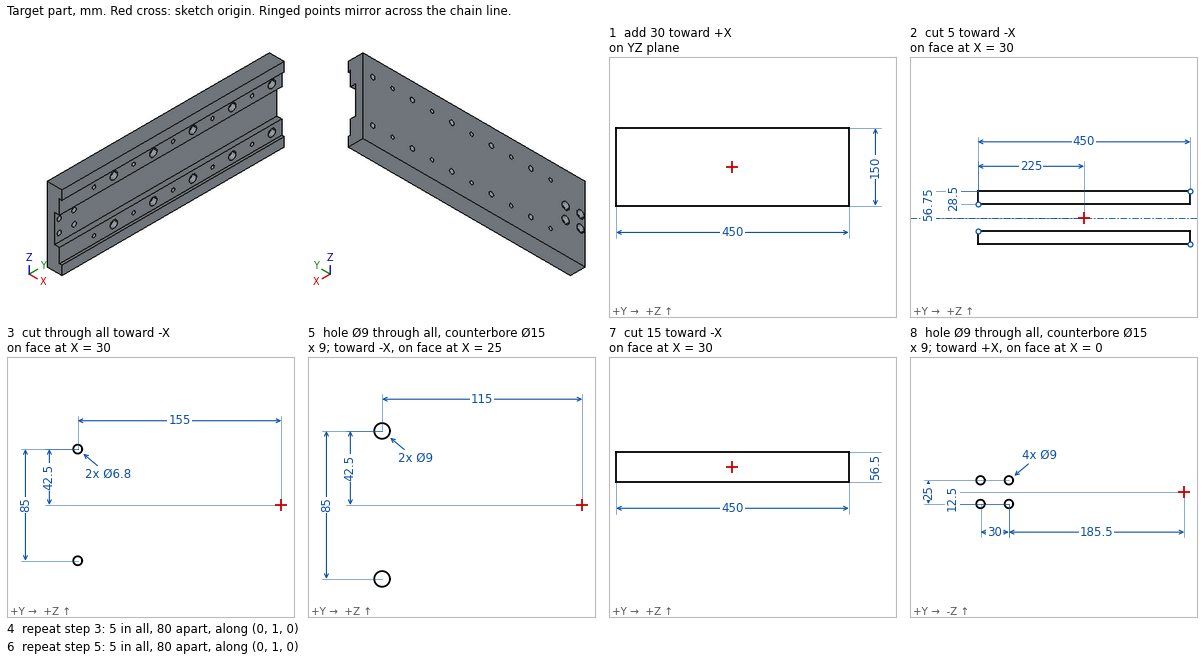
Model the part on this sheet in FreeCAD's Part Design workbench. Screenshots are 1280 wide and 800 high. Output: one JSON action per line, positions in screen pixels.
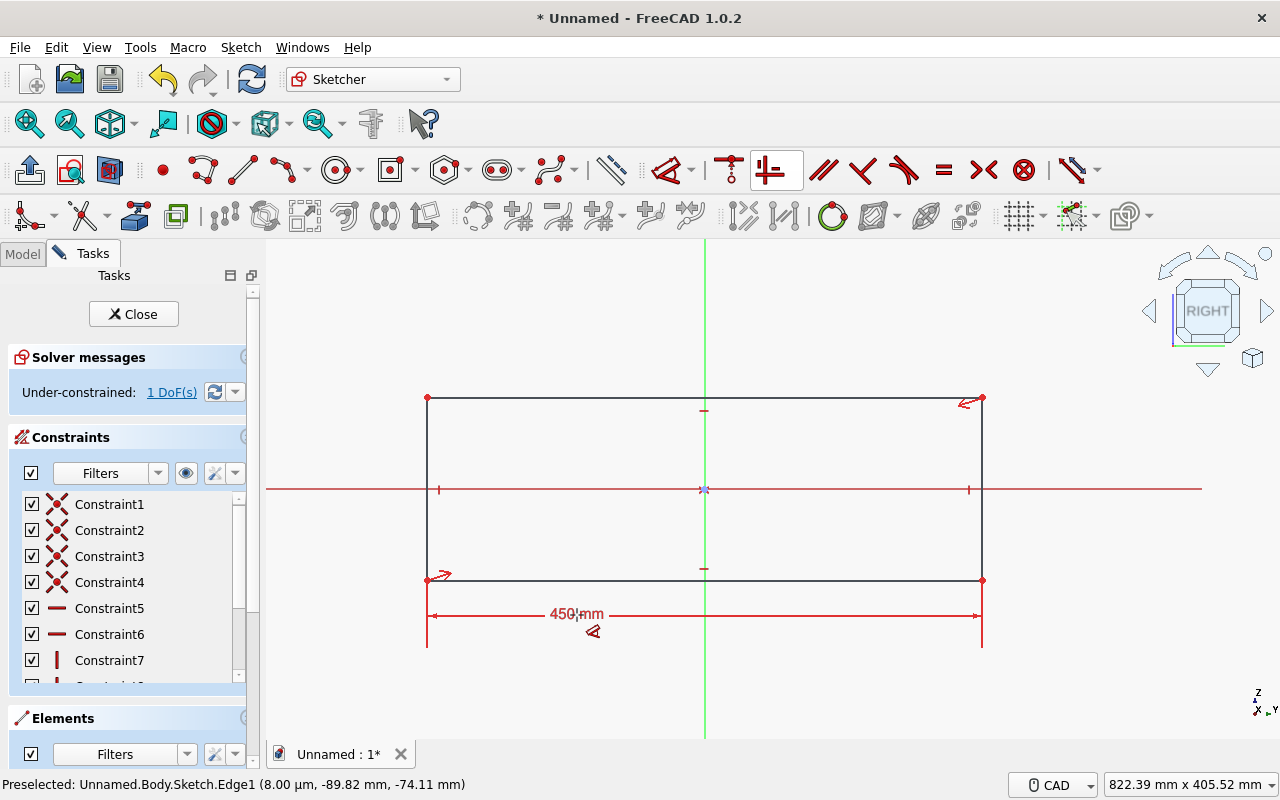
{"action": "left_click", "coordinate": [982, 526]}
{"action": "left_click", "coordinate": [1016, 447]}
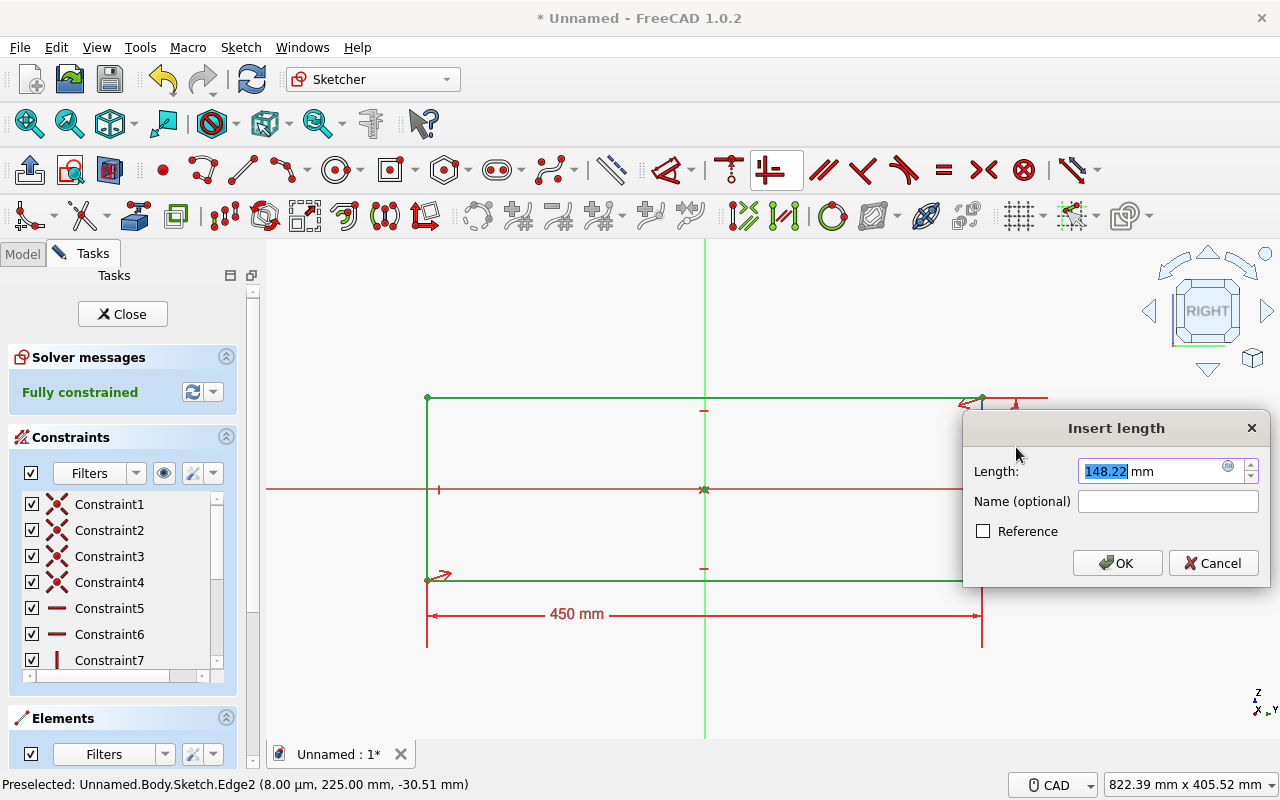
{"action": "type", "text": "150"}
{"action": "key", "text": "Return"}
{"action": "key", "text": "Escape"}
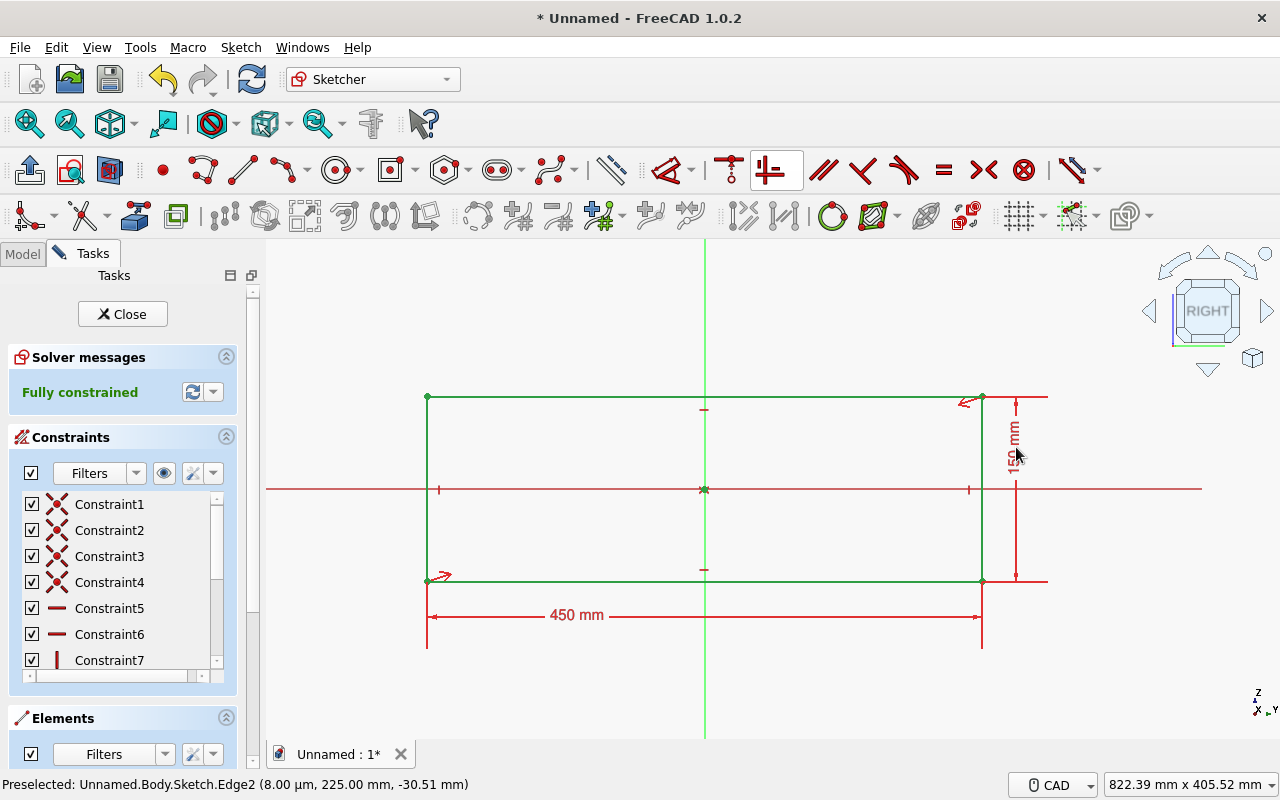
{"action": "left_click", "coordinate": [123, 314]}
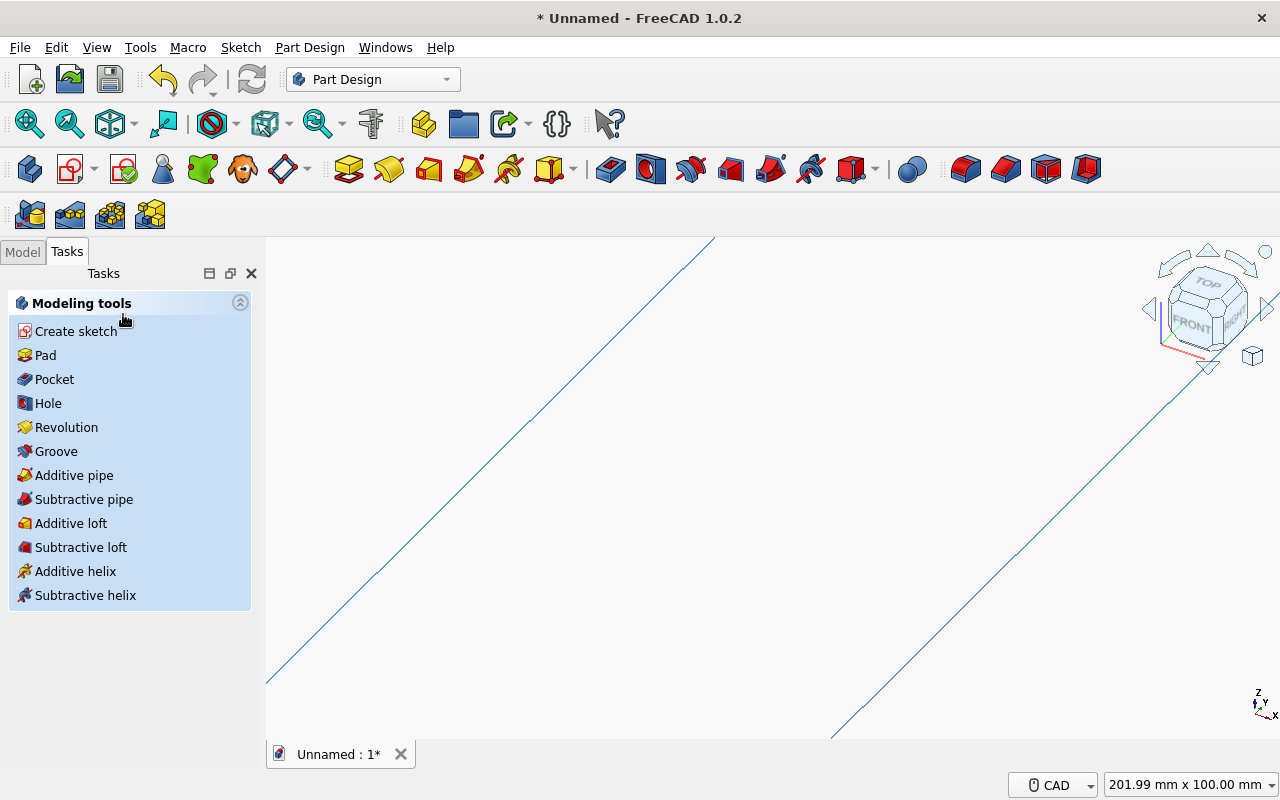
{"action": "left_click", "coordinate": [350, 170]}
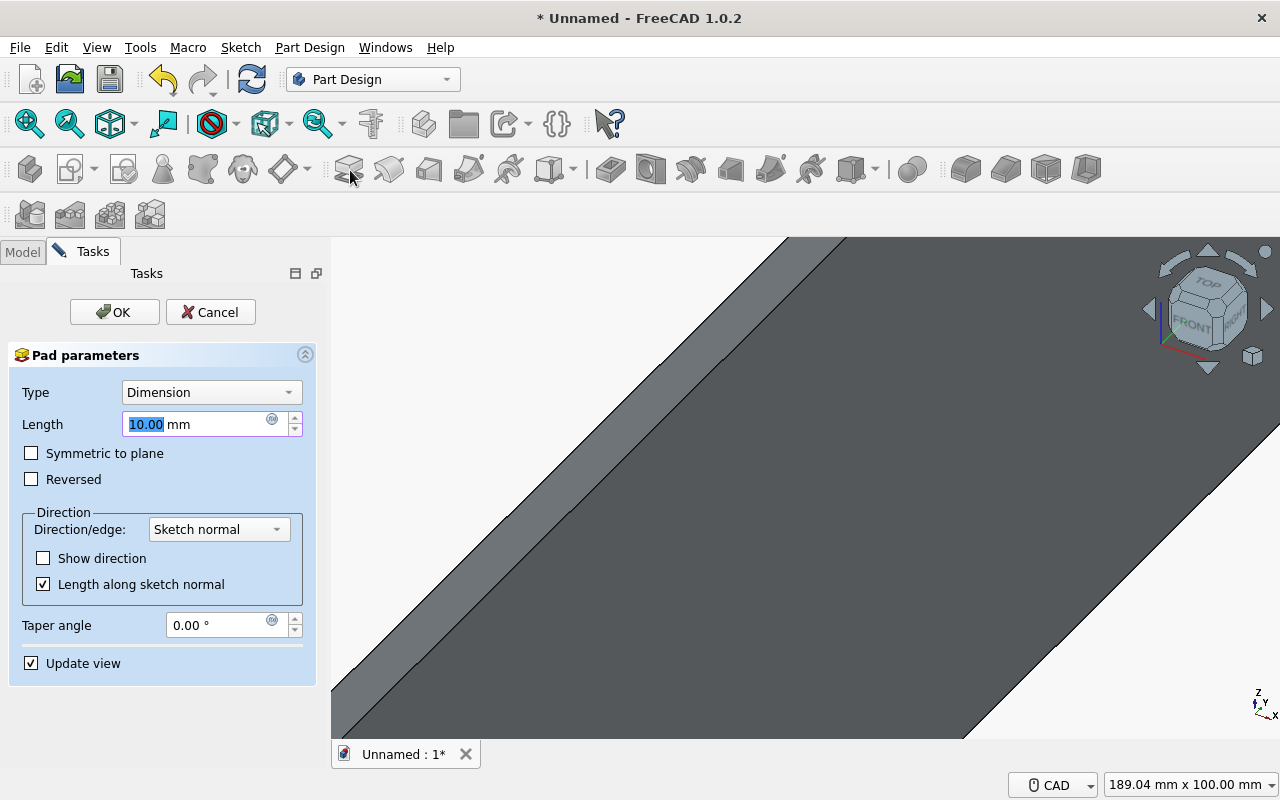
{"action": "type", "text": "30"}
{"action": "key", "text": "Tab"}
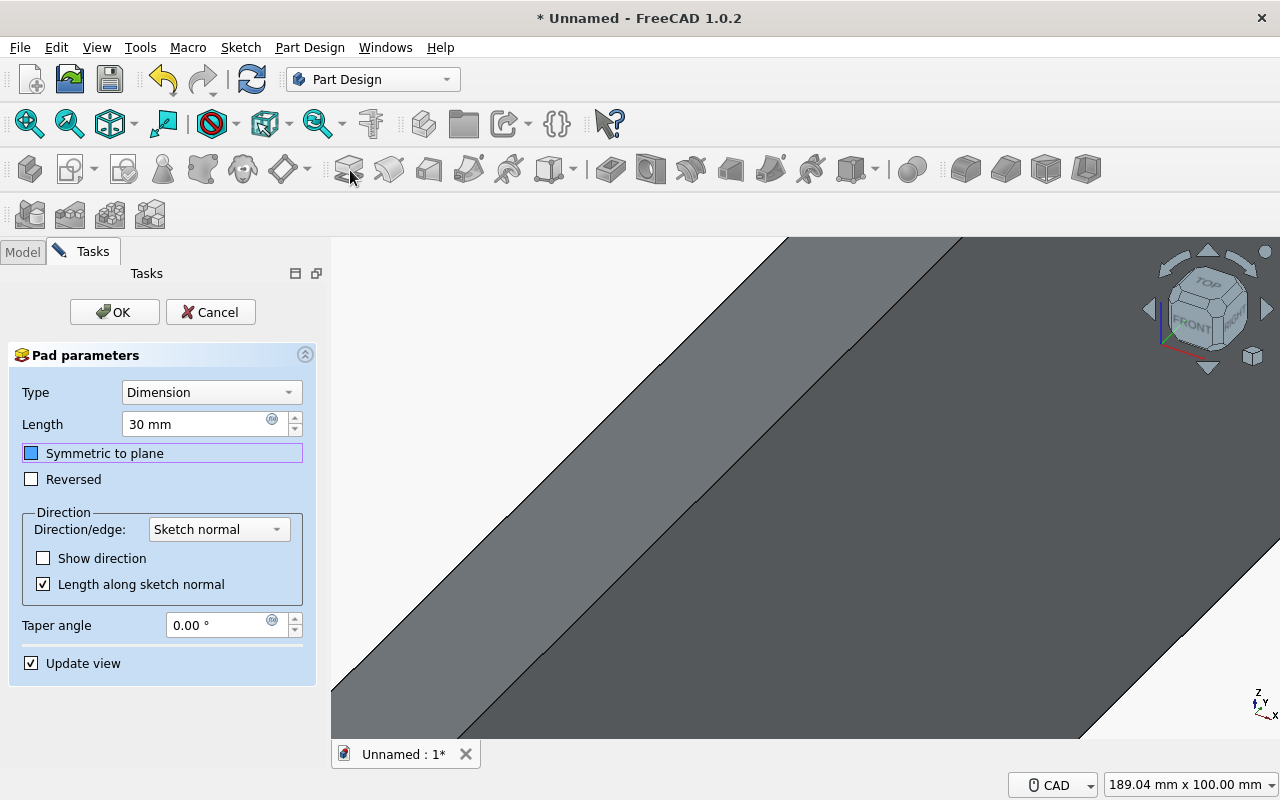
{"action": "left_click", "coordinate": [115, 312]}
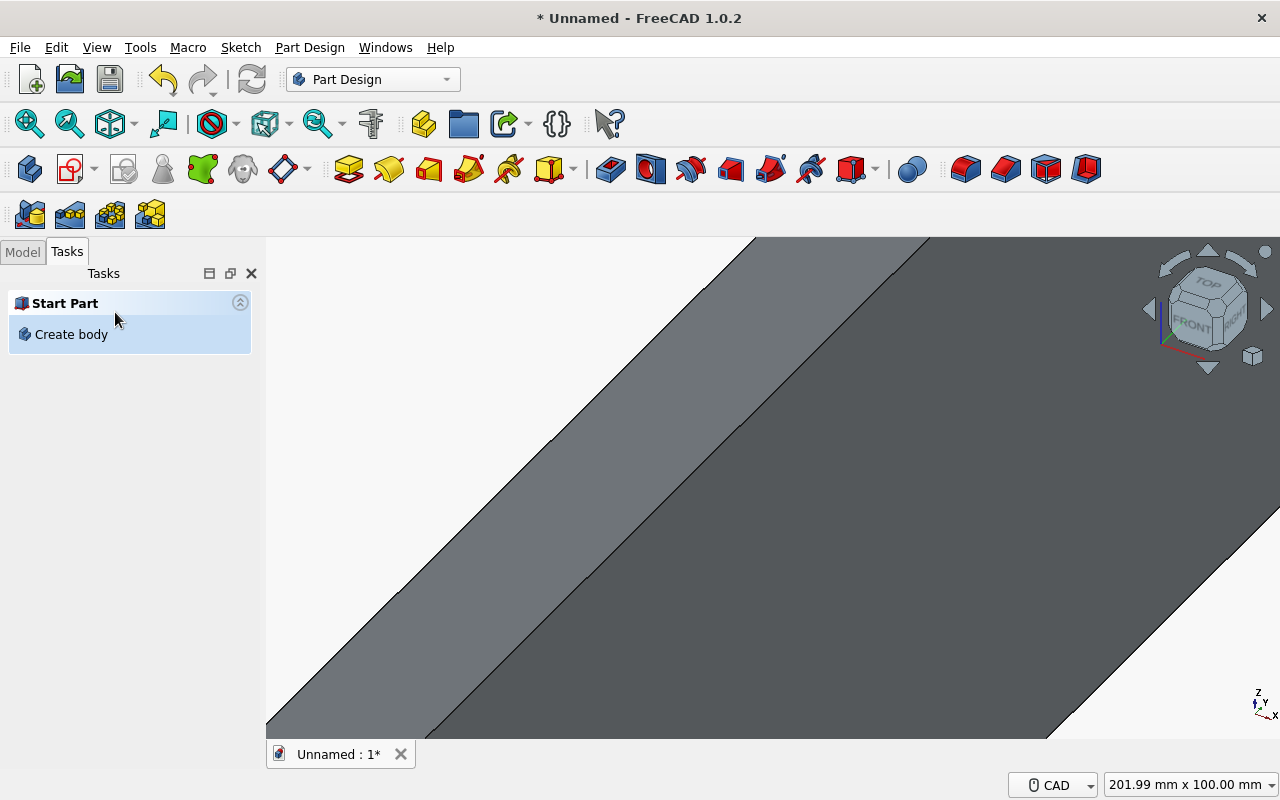
{"action": "left_click", "coordinate": [30, 124]}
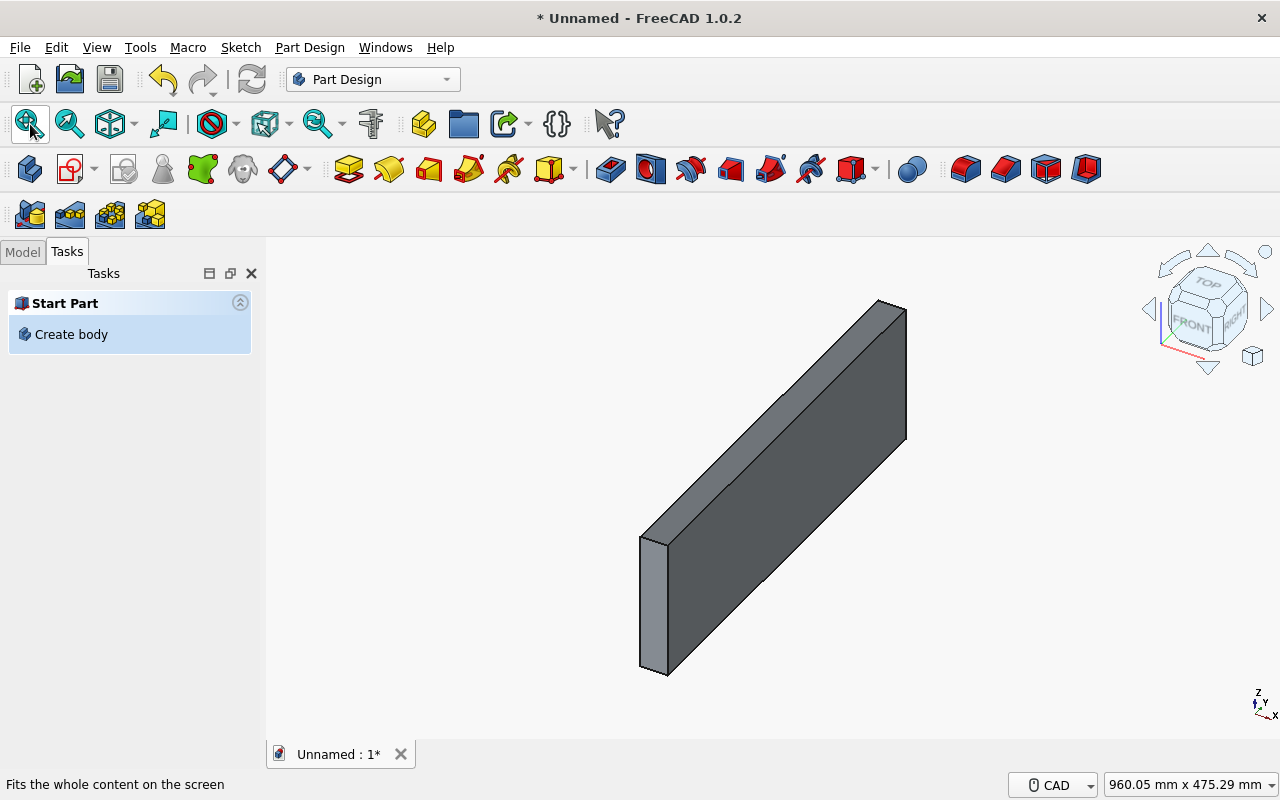
{"action": "left_click", "coordinate": [855, 424]}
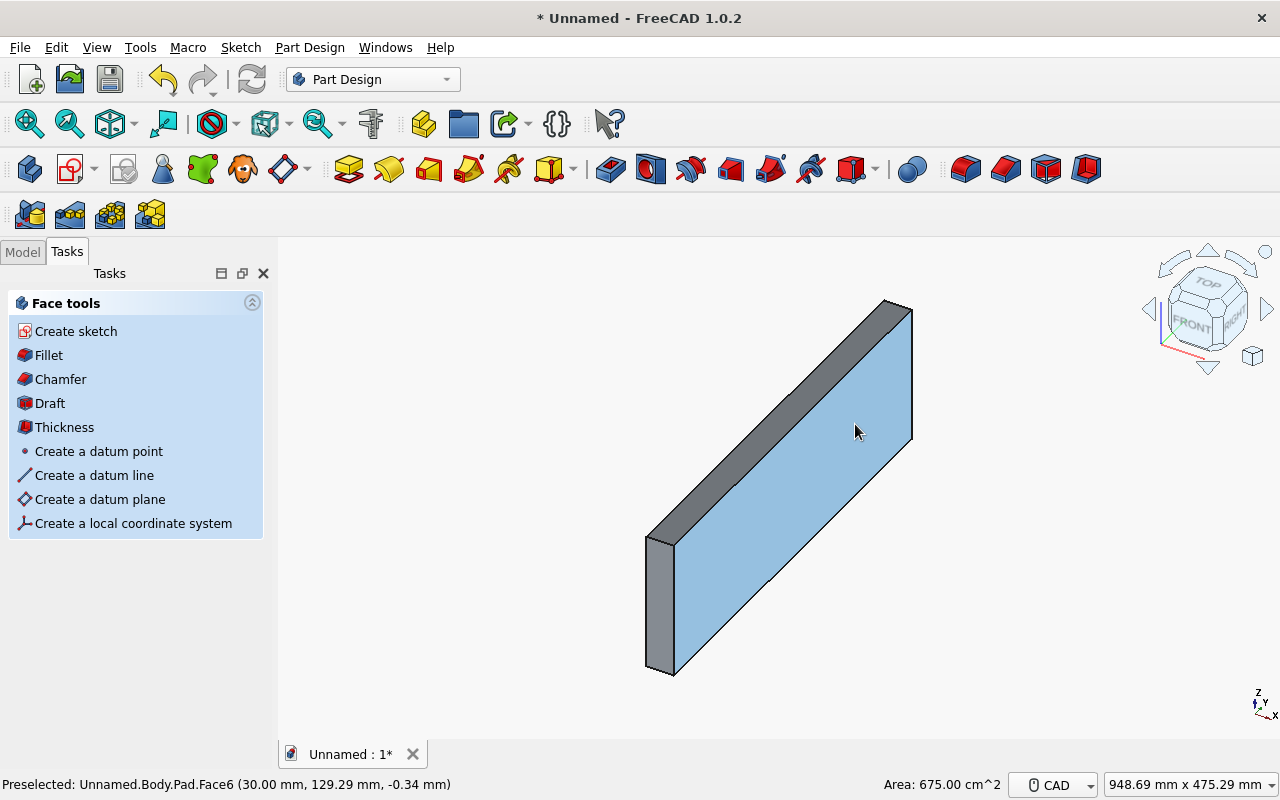
{"action": "left_click", "coordinate": [70, 170]}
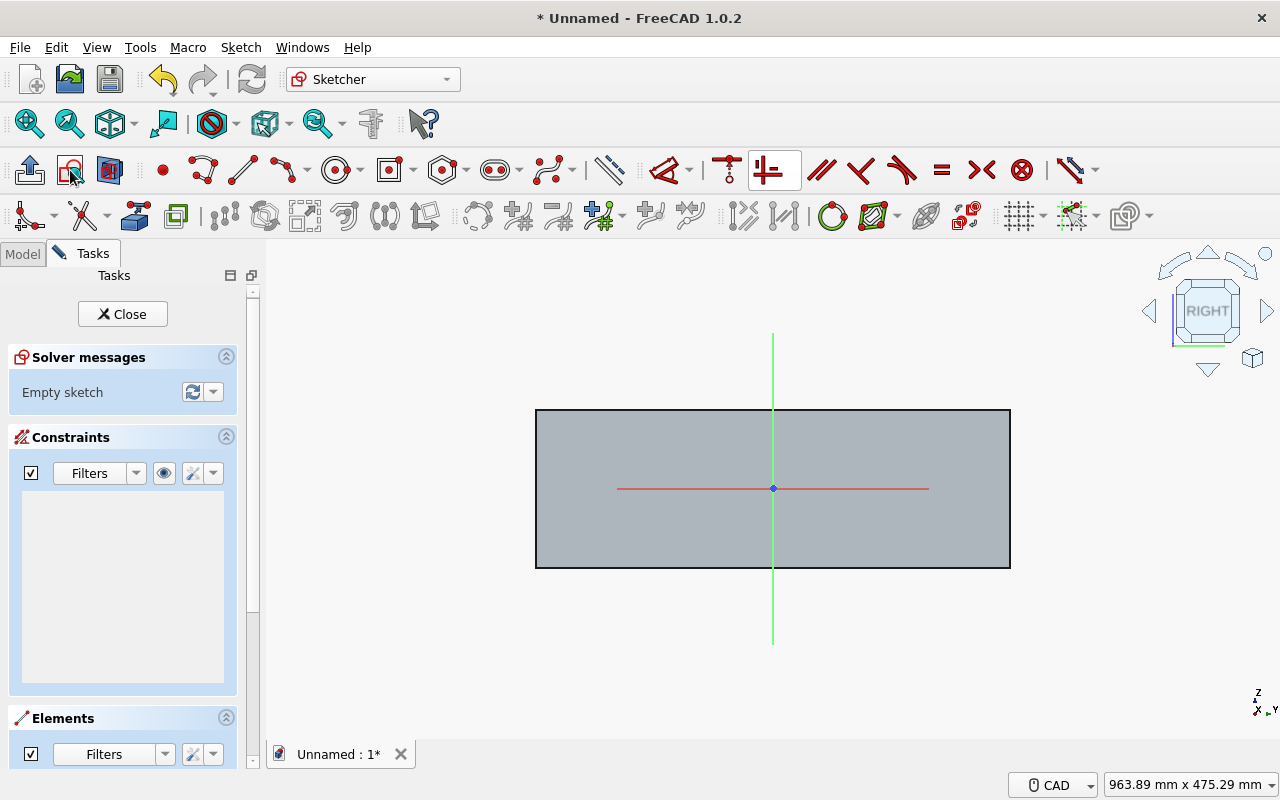
{"action": "key", "text": "g r"}